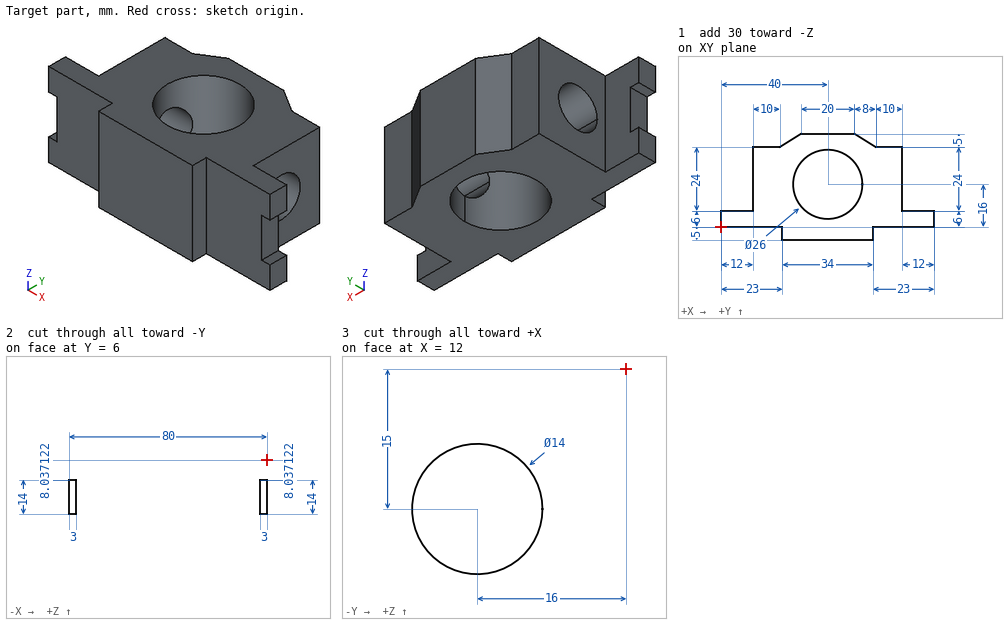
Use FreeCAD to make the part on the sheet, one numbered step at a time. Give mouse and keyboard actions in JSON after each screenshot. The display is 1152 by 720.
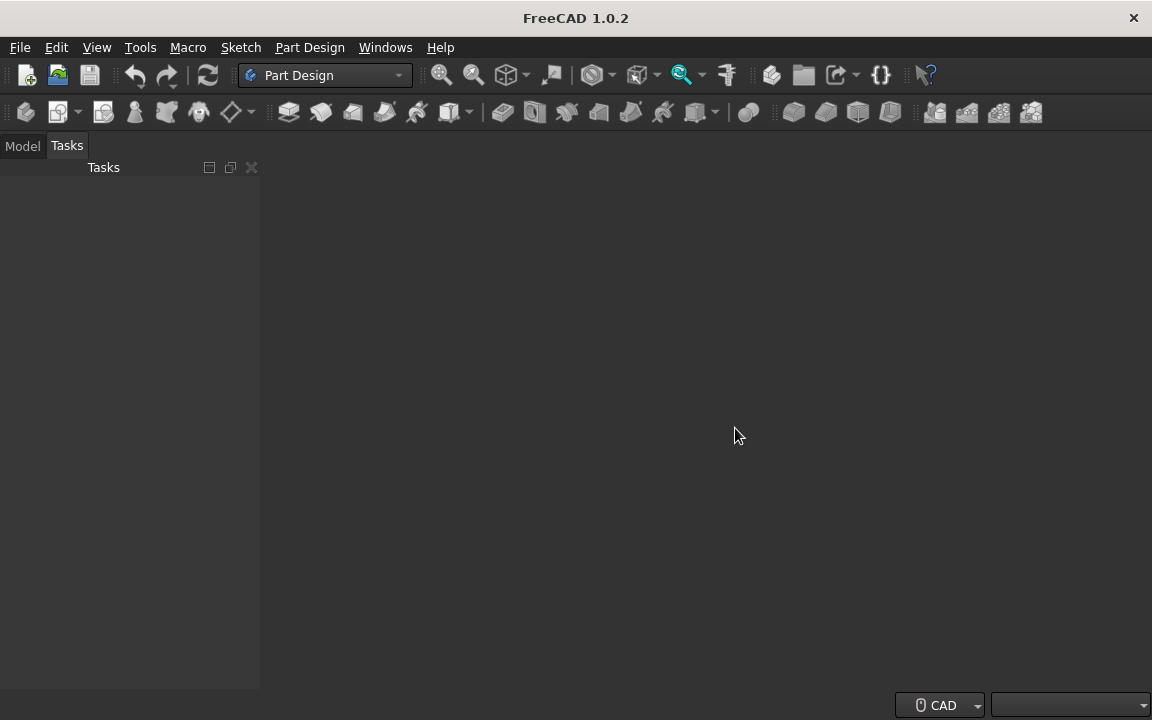
{"action": "key", "text": "ctrl+n"}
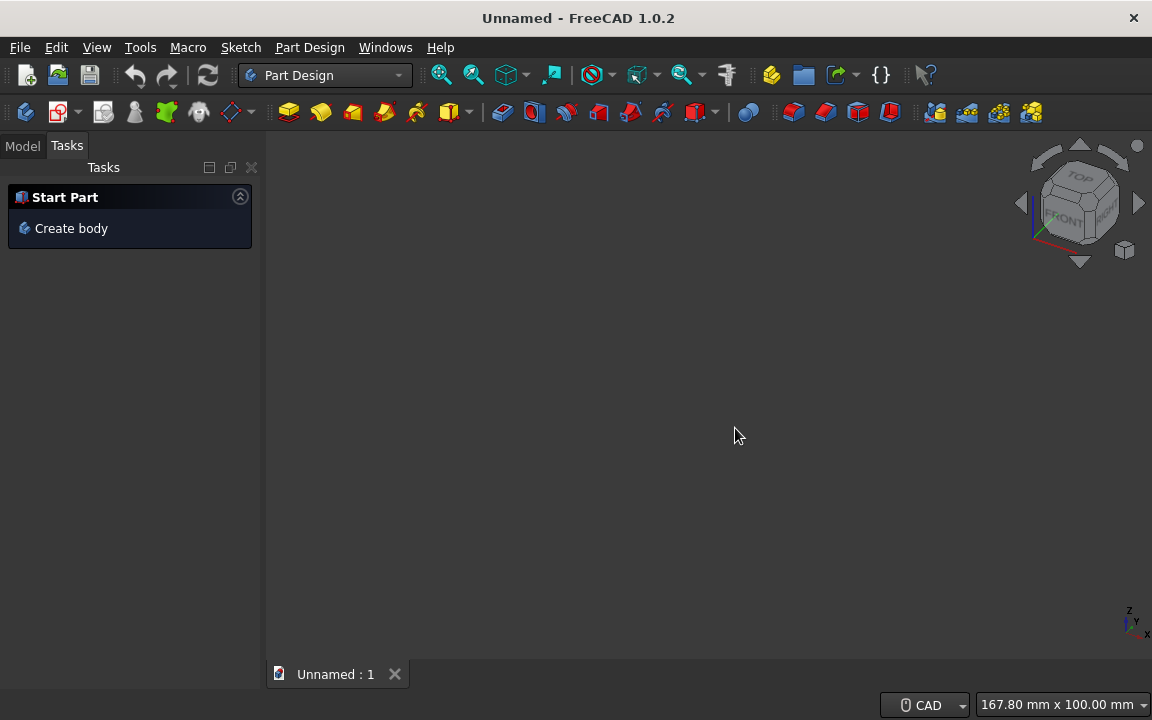
{"action": "left_click", "coordinate": [58, 112]}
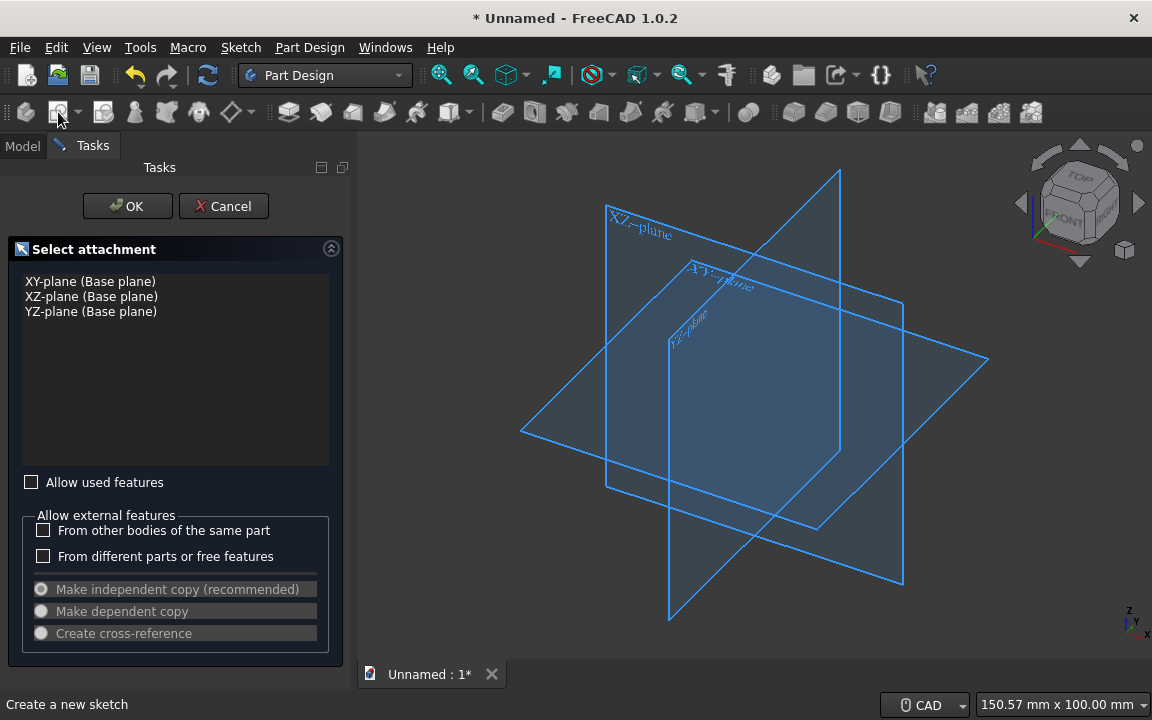
{"action": "left_click", "coordinate": [82, 282]}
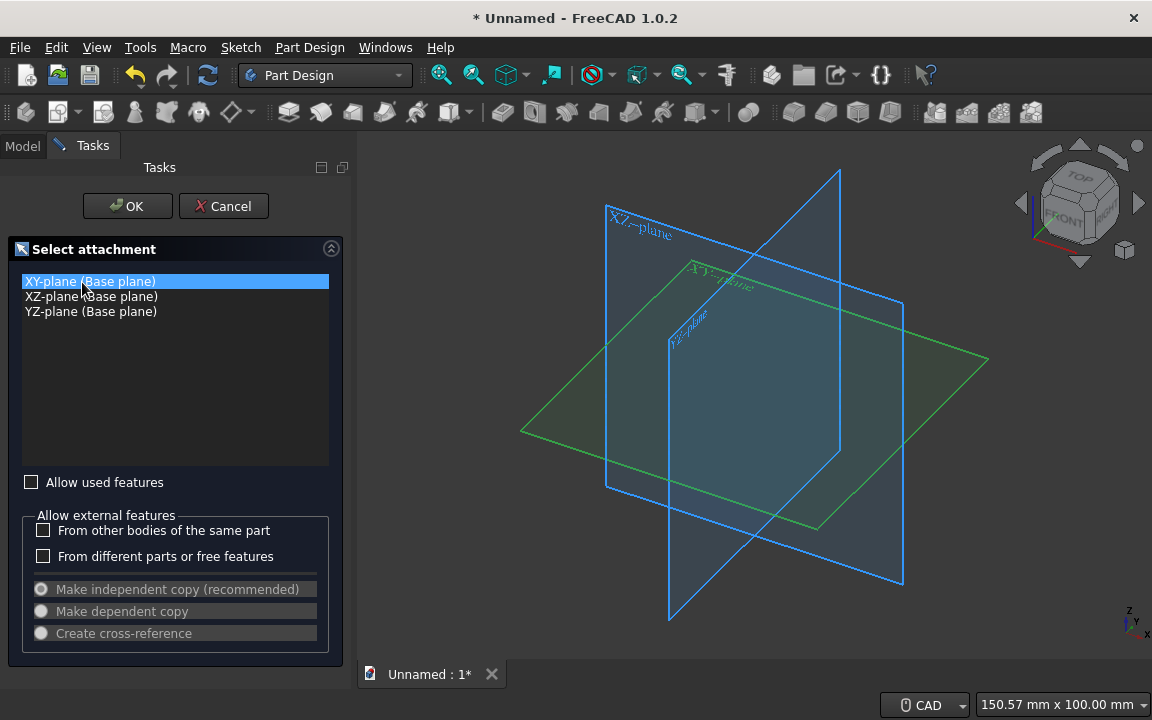
{"action": "left_click", "coordinate": [128, 206]}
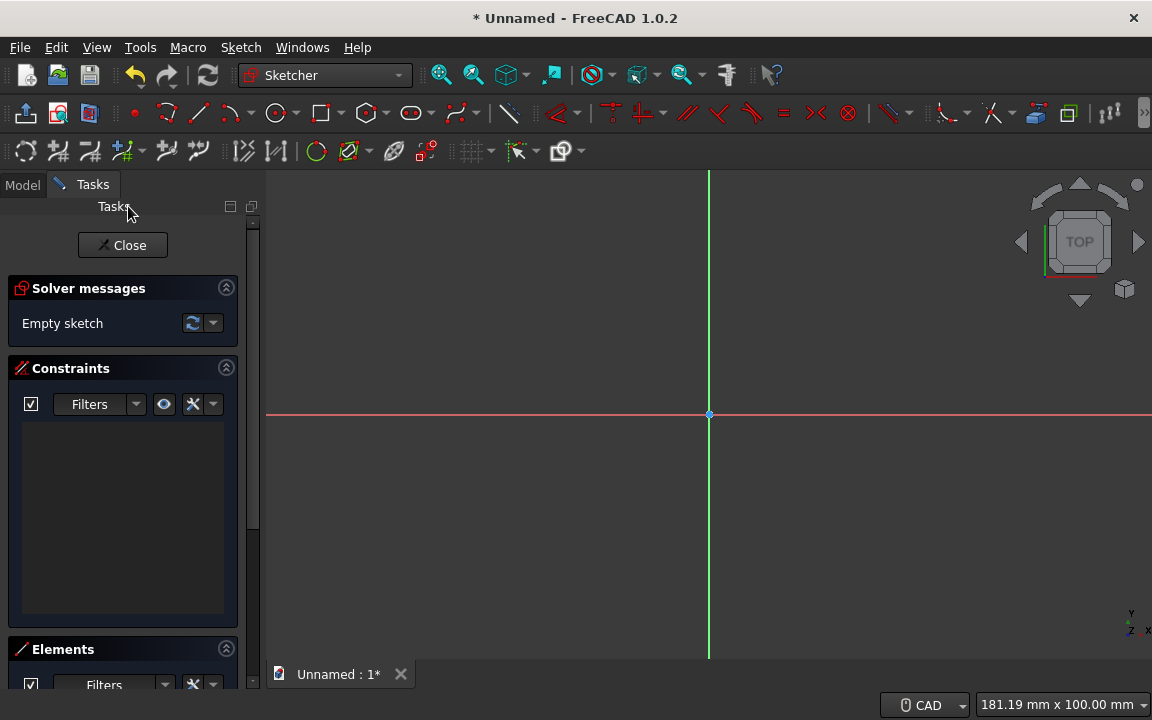
{"action": "scroll", "coordinate": [294, 631], "scroll_direction": "down", "scroll_amount": 1}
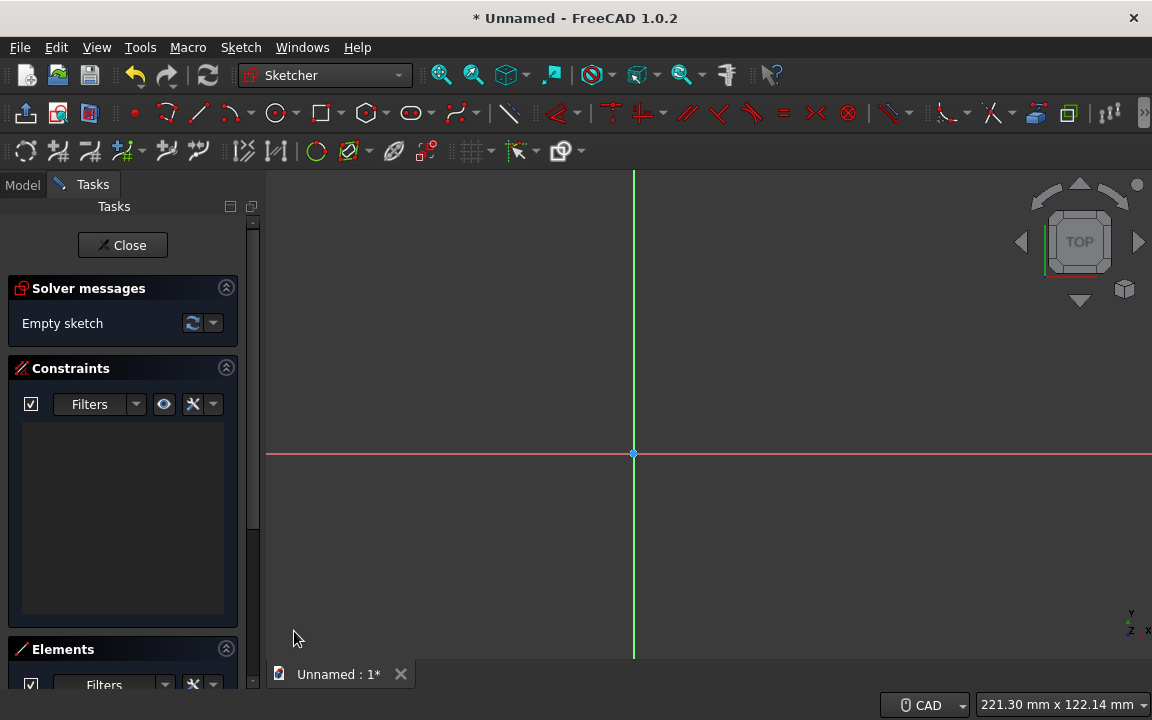
{"action": "scroll", "coordinate": [987, 352], "scroll_direction": "up", "scroll_amount": 2}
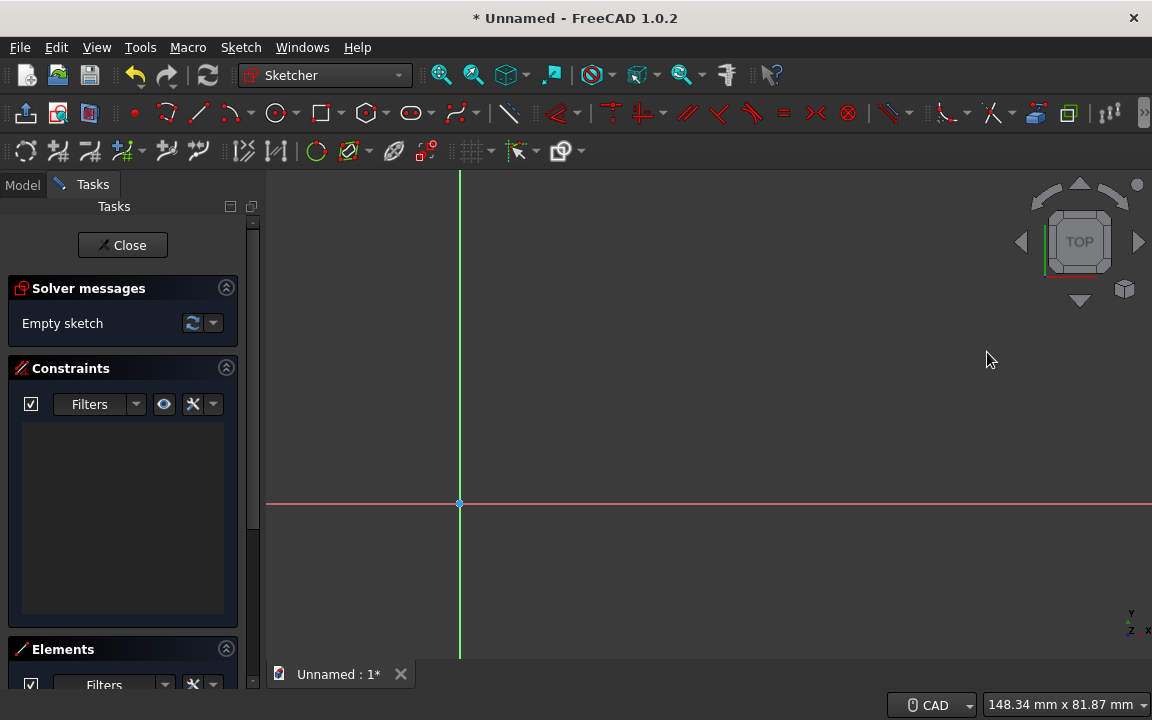
{"action": "key", "text": "g m"}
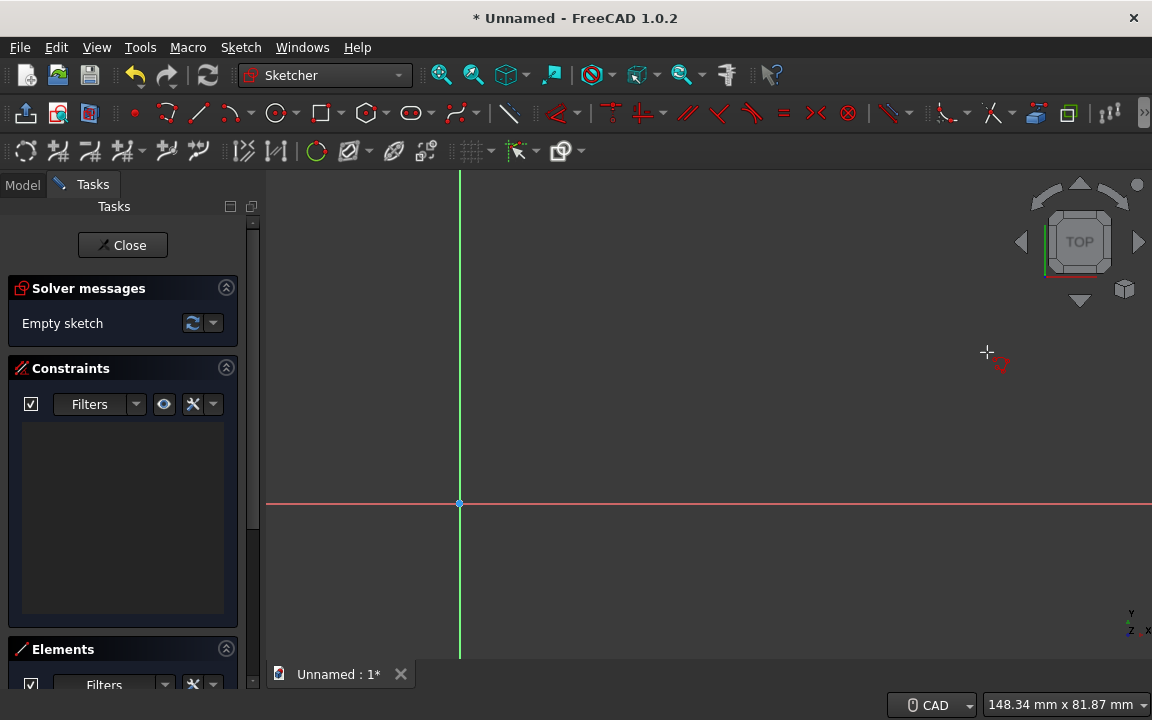
{"action": "left_click", "coordinate": [460, 504]}
{"action": "left_click", "coordinate": [597, 495]}
{"action": "left_click", "coordinate": [597, 534]}
{"action": "left_click", "coordinate": [800, 534]}
{"action": "left_click", "coordinate": [800, 504]}
{"action": "left_click", "coordinate": [937, 495]}
{"action": "left_click", "coordinate": [937, 468]}
{"action": "left_click", "coordinate": [866, 468]}
{"action": "left_click", "coordinate": [866, 325]}
{"action": "left_click", "coordinate": [806, 325]}
{"action": "left_click", "coordinate": [758, 295]}
{"action": "left_click", "coordinate": [639, 295]}
{"action": "left_click", "coordinate": [591, 325]}
{"action": "left_click", "coordinate": [531, 325]}
{"action": "left_click", "coordinate": [531, 468]}
{"action": "left_click", "coordinate": [469, 468]}
{"action": "left_click", "coordinate": [460, 504]}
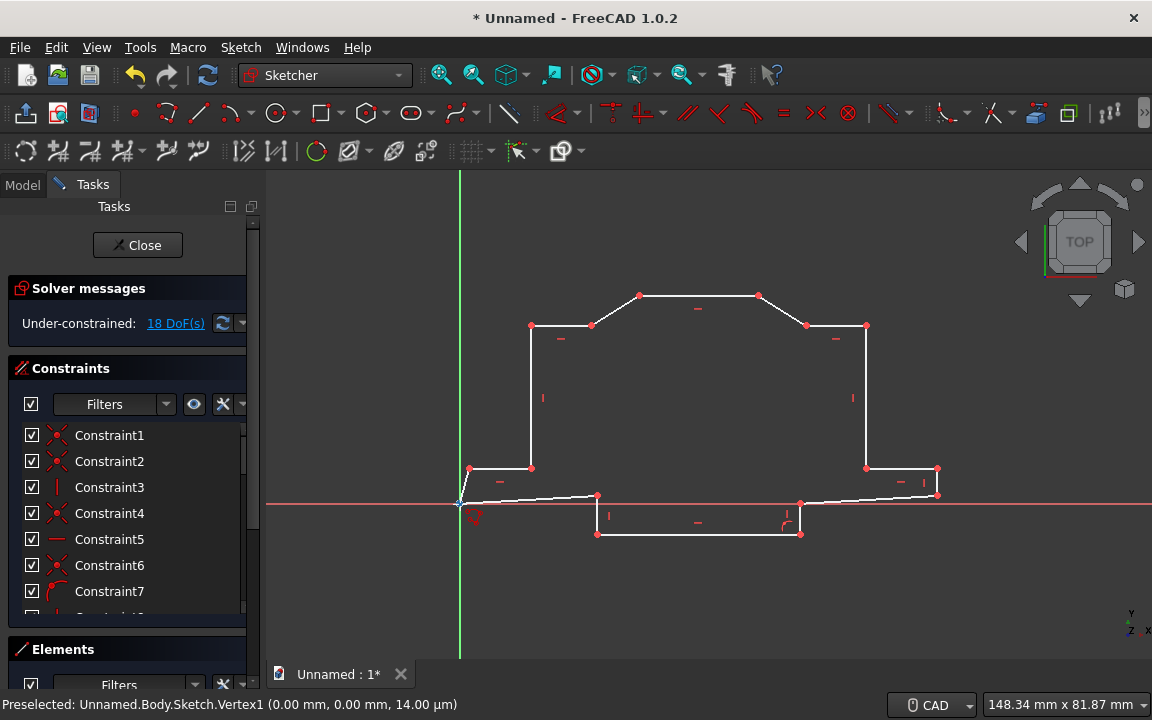
{"action": "key", "text": "g c"}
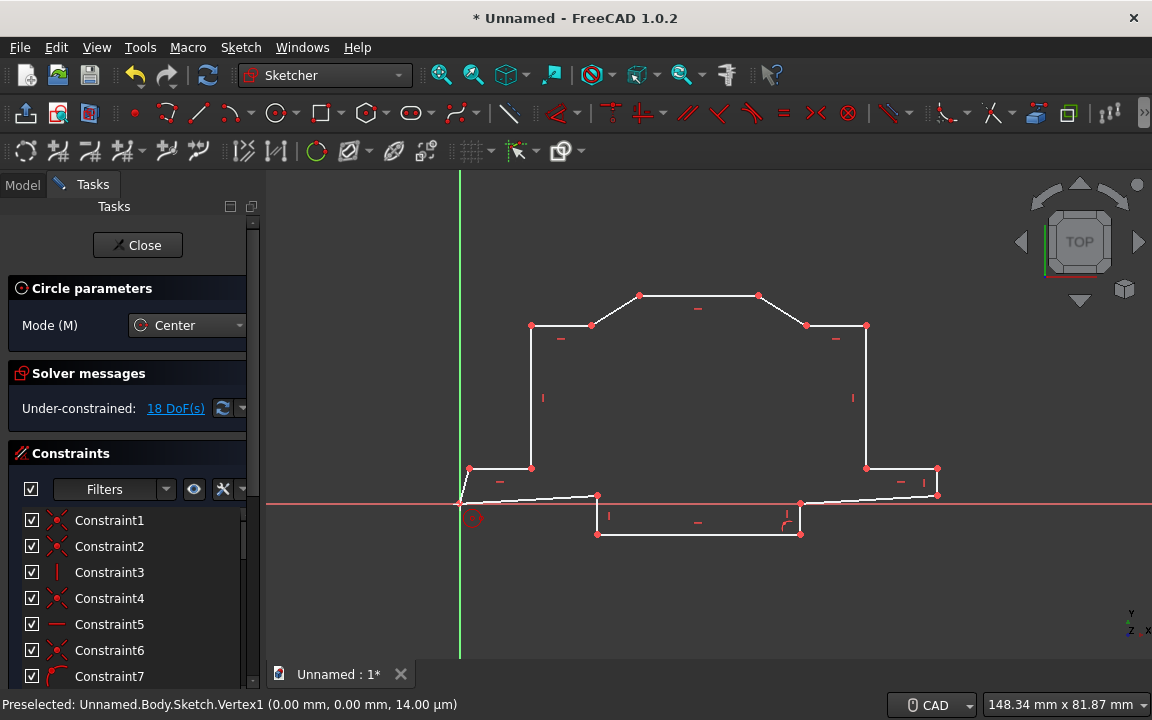
{"action": "left_click", "coordinate": [699, 408]}
{"action": "left_click", "coordinate": [753, 353]}
{"action": "key", "text": "Escape"}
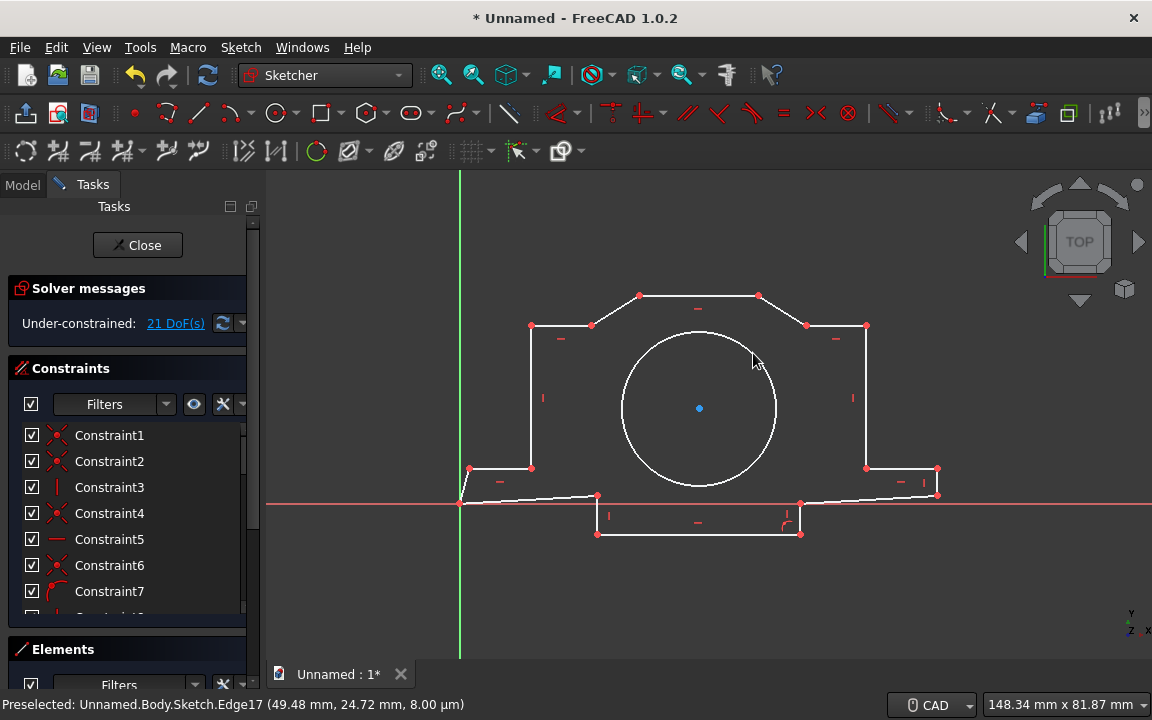
{"action": "left_click", "coordinate": [501, 502]}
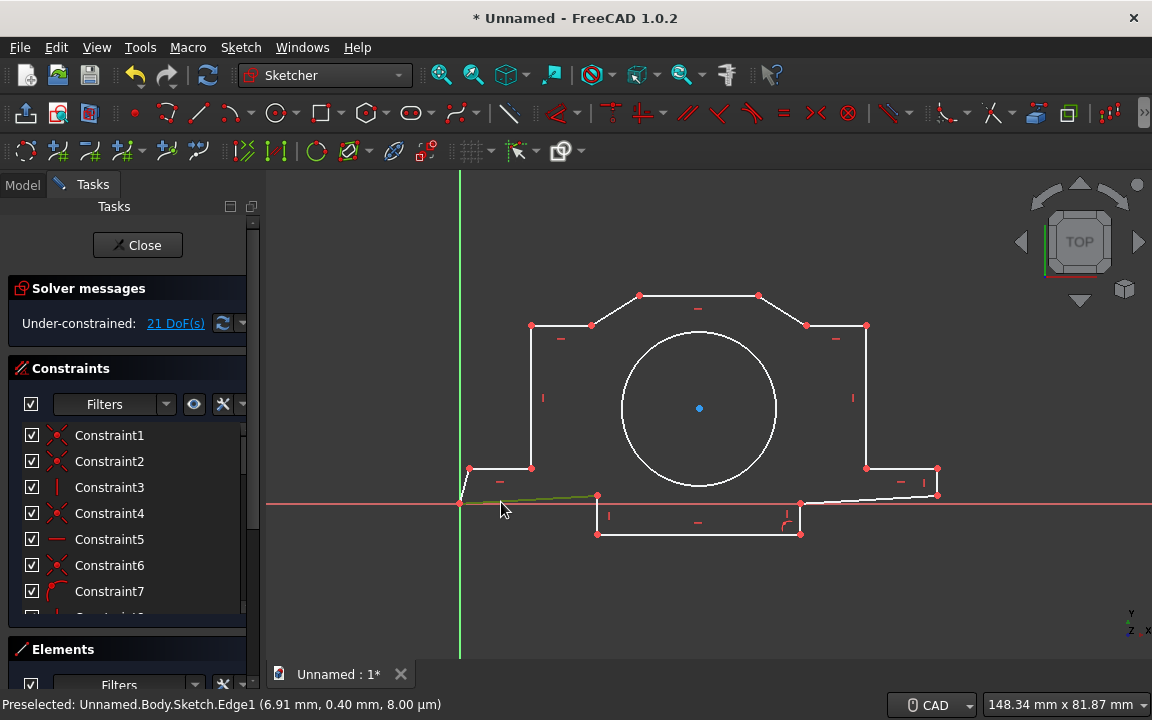
{"action": "key", "text": "h"}